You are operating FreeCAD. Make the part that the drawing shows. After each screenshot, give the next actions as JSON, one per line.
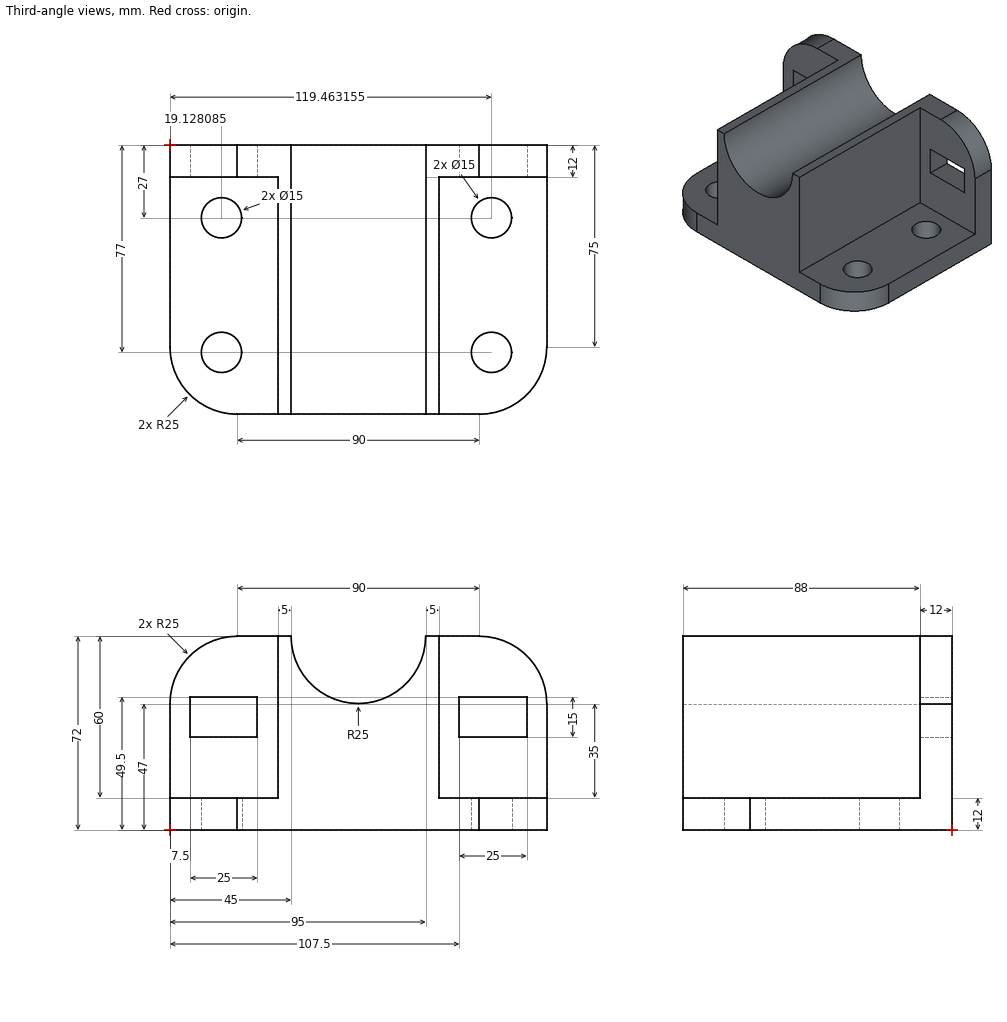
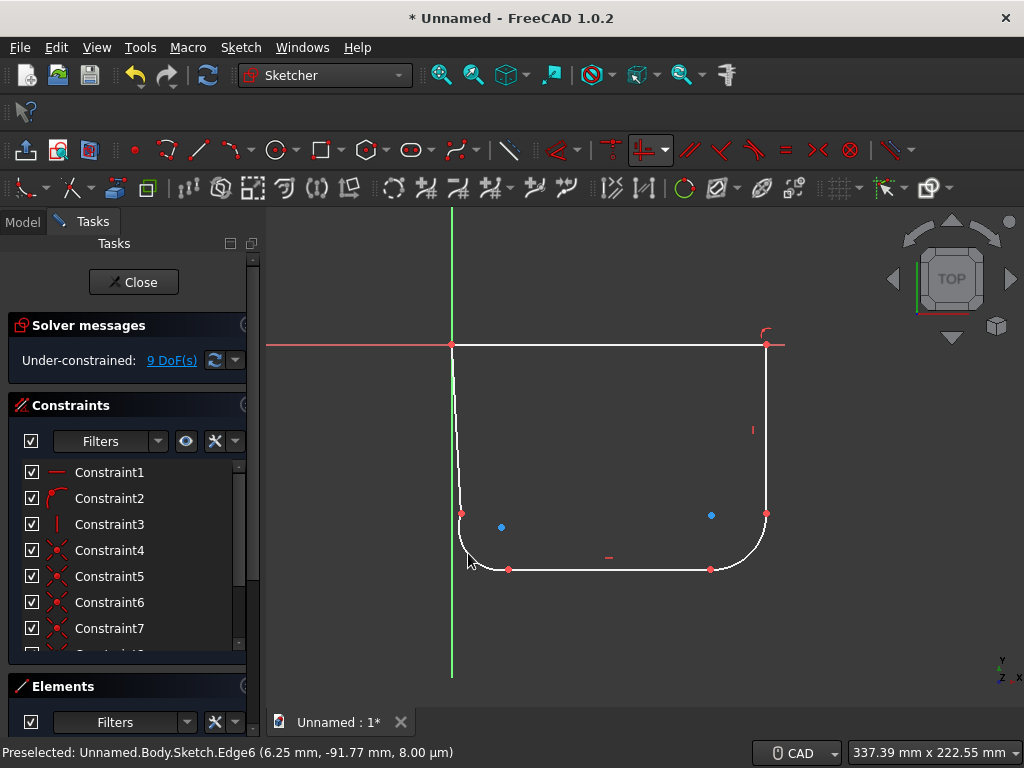
{"action": "left_click", "coordinate": [569, 570]}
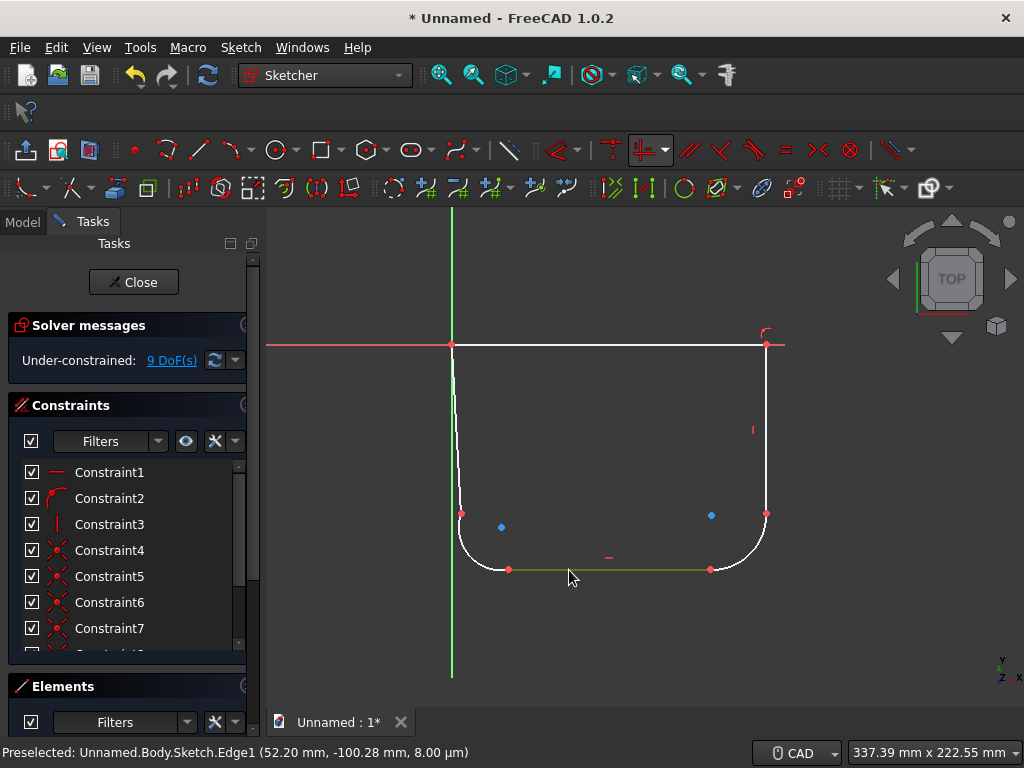
{"action": "left_click", "coordinate": [736, 564]}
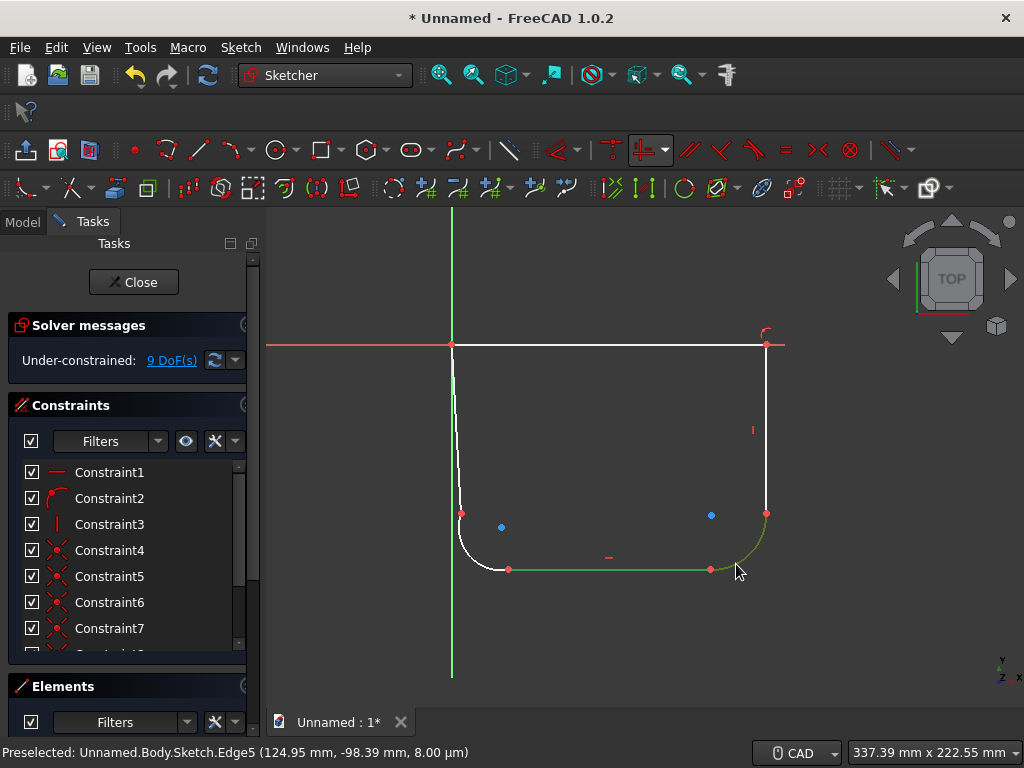
{"action": "key", "text": "t"}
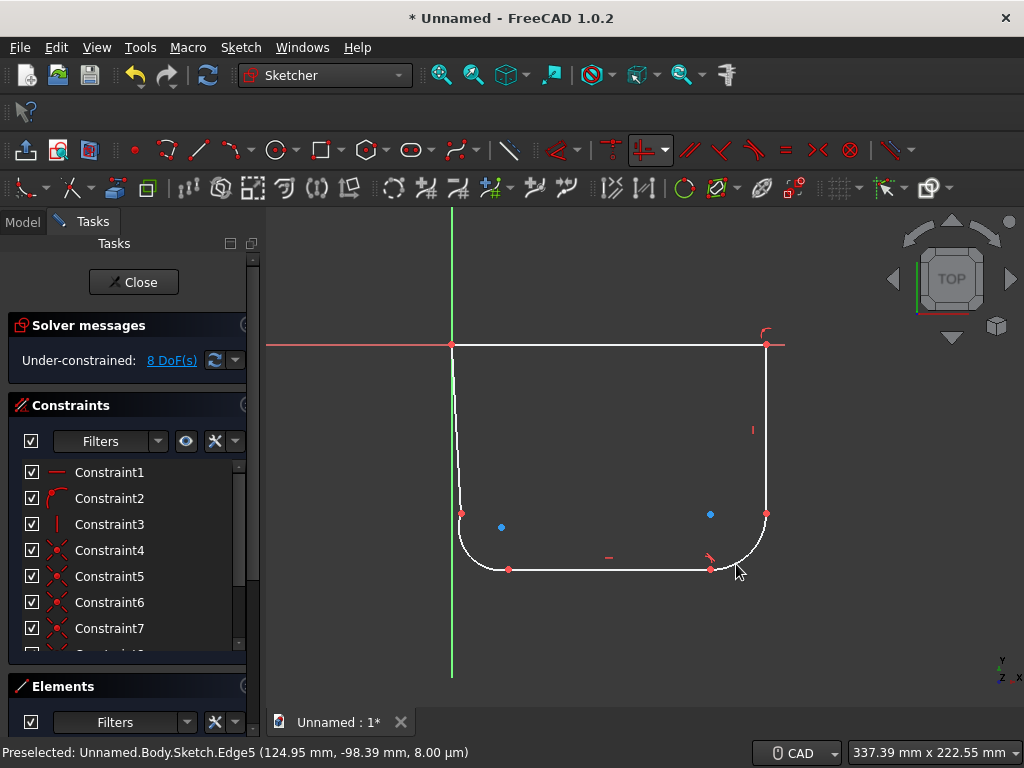
{"action": "left_click", "coordinate": [569, 570]}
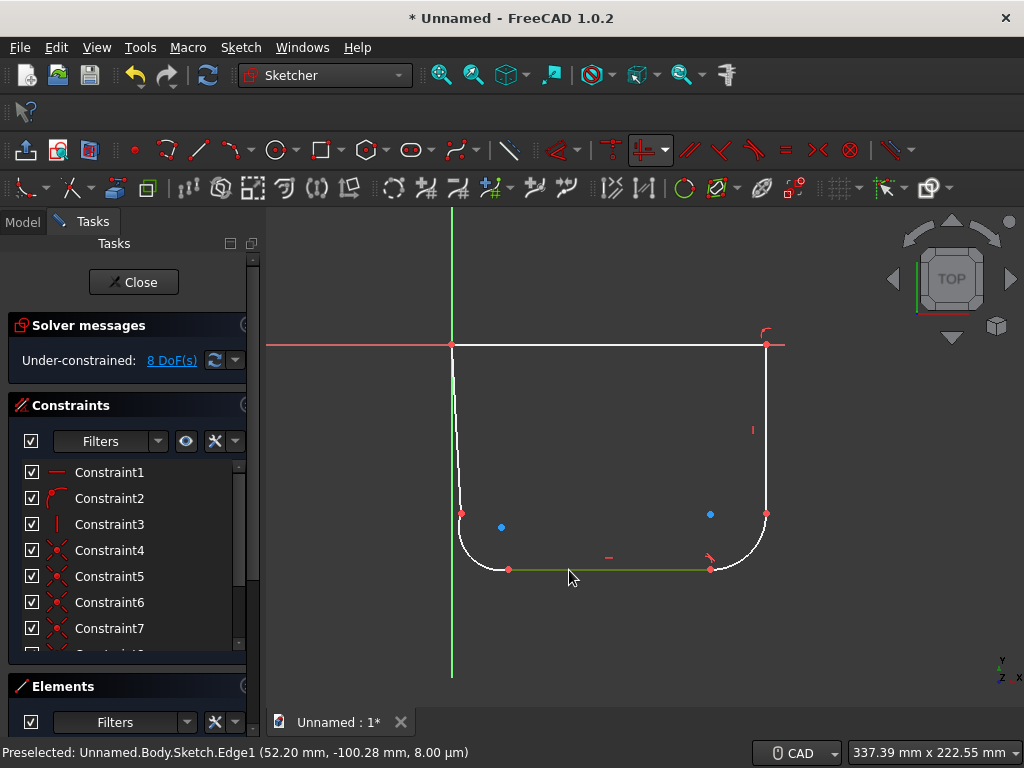
{"action": "left_click", "coordinate": [483, 566]}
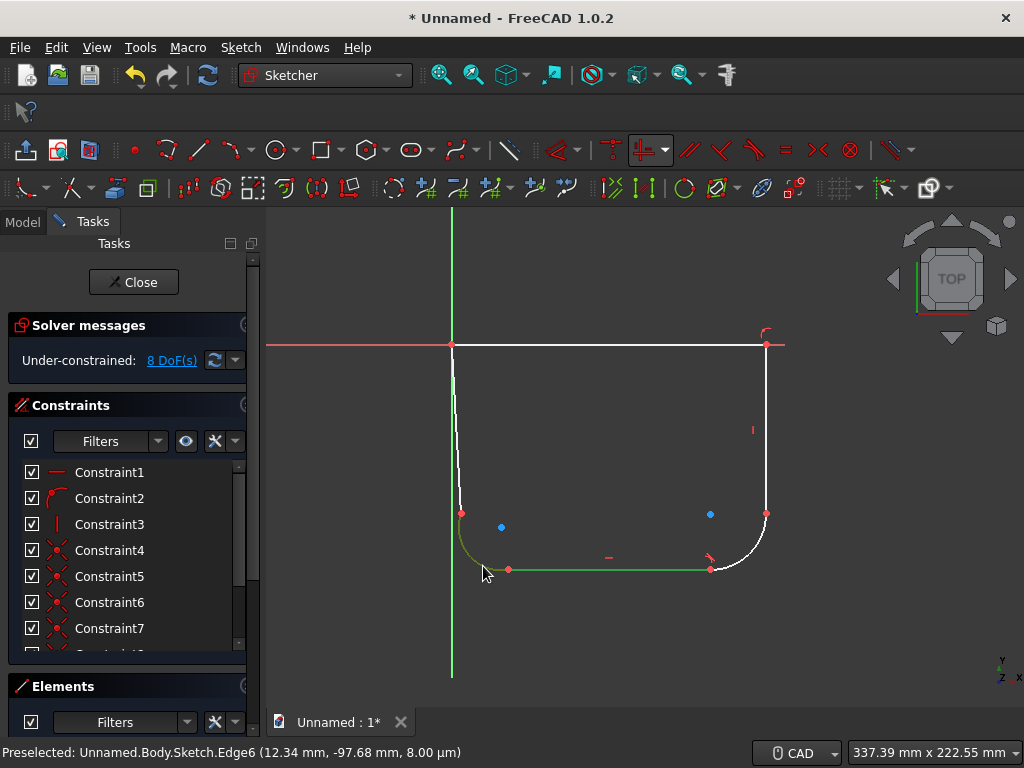
{"action": "key", "text": "t"}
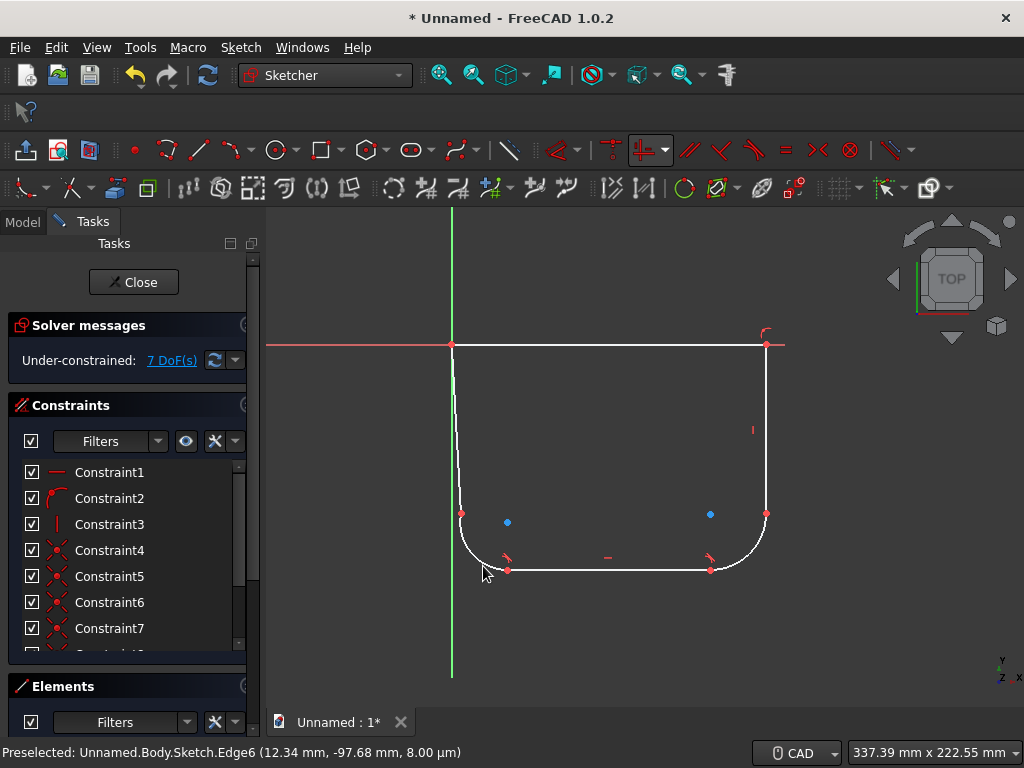
{"action": "left_click", "coordinate": [766, 463]}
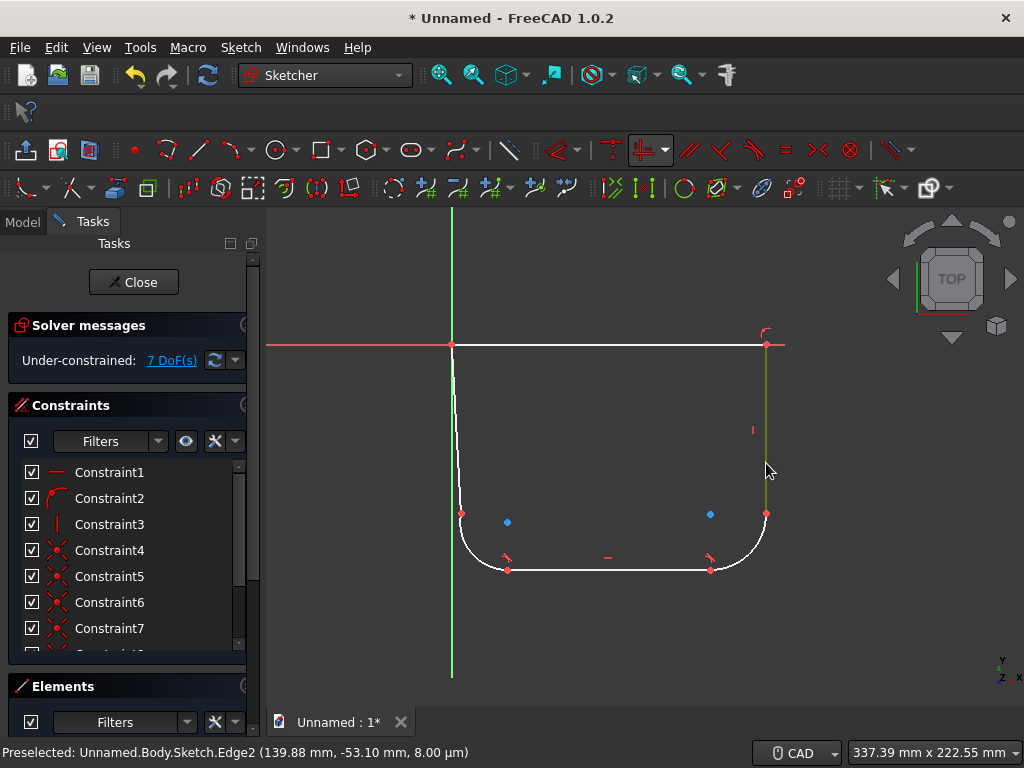
{"action": "left_click", "coordinate": [735, 564]}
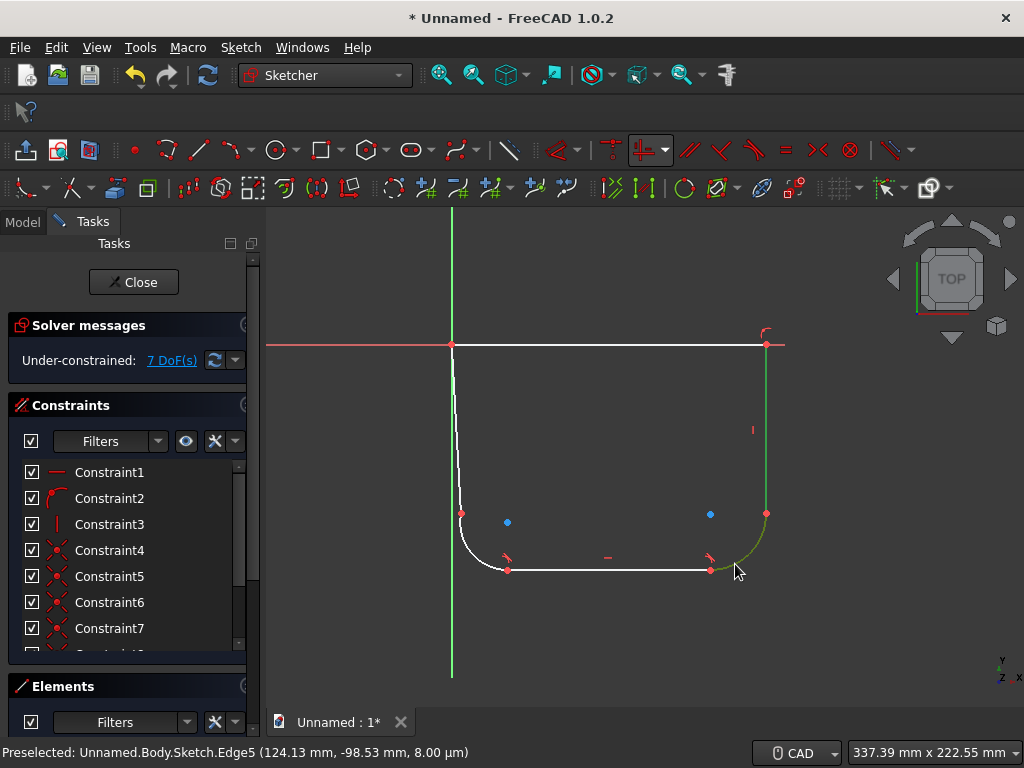
{"action": "left_click", "coordinate": [754, 150]}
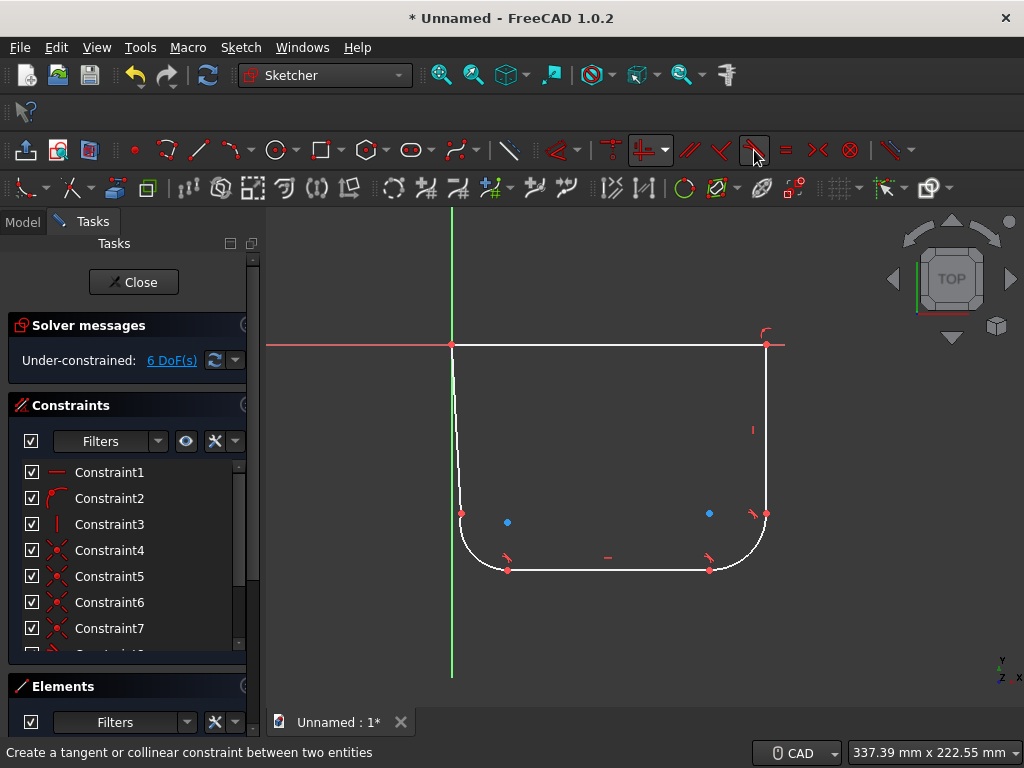
{"action": "left_click", "coordinate": [455, 395]}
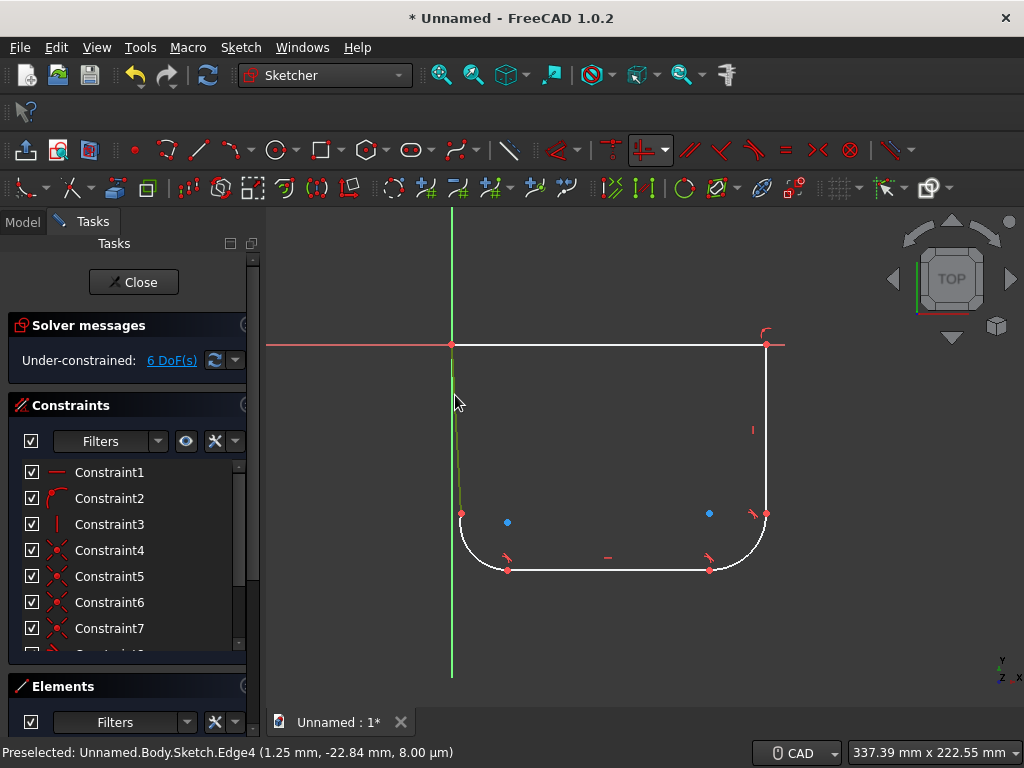
{"action": "left_click", "coordinate": [463, 539]}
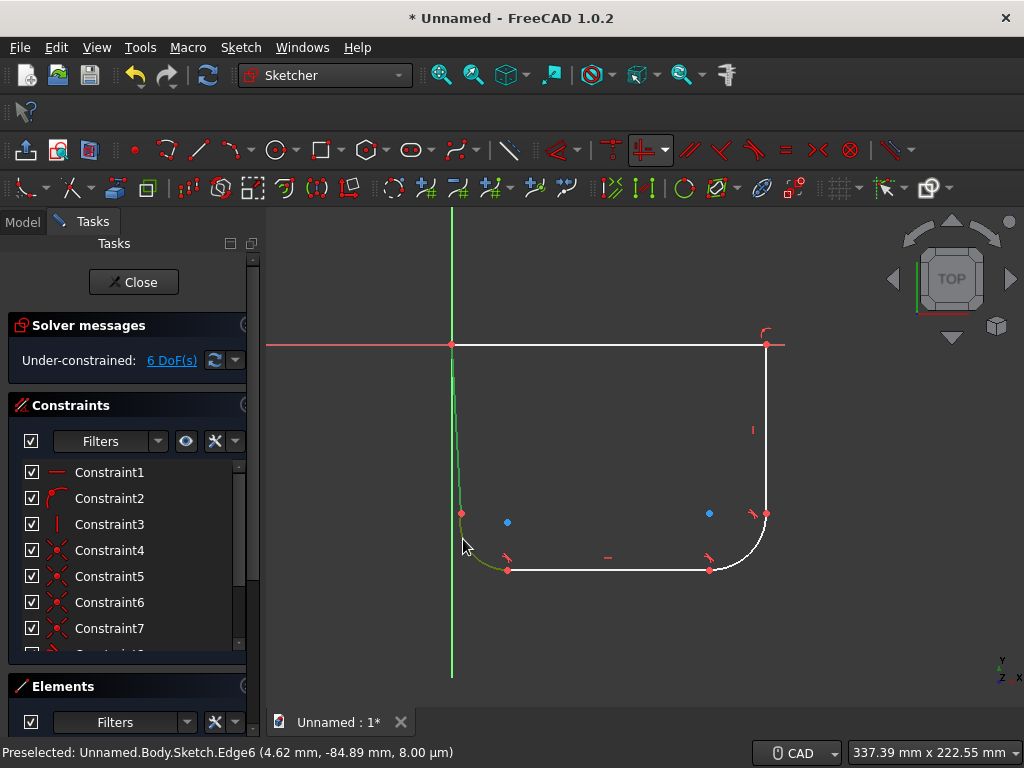
{"action": "left_click", "coordinate": [754, 150]}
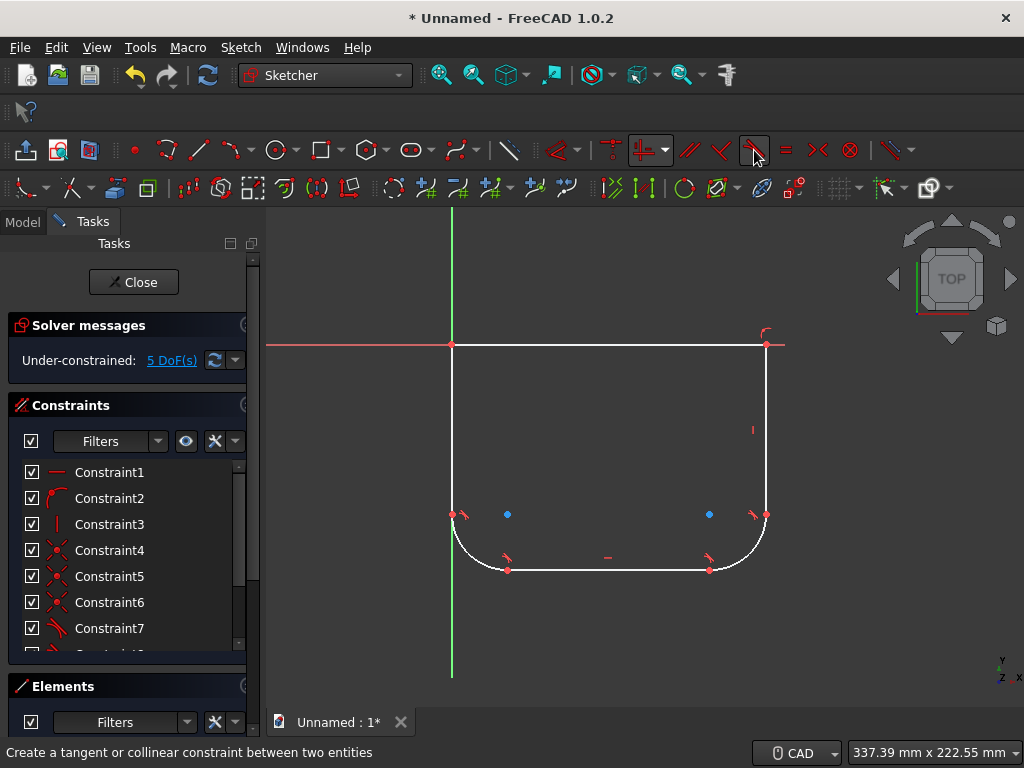
{"action": "left_click", "coordinate": [452, 396]}